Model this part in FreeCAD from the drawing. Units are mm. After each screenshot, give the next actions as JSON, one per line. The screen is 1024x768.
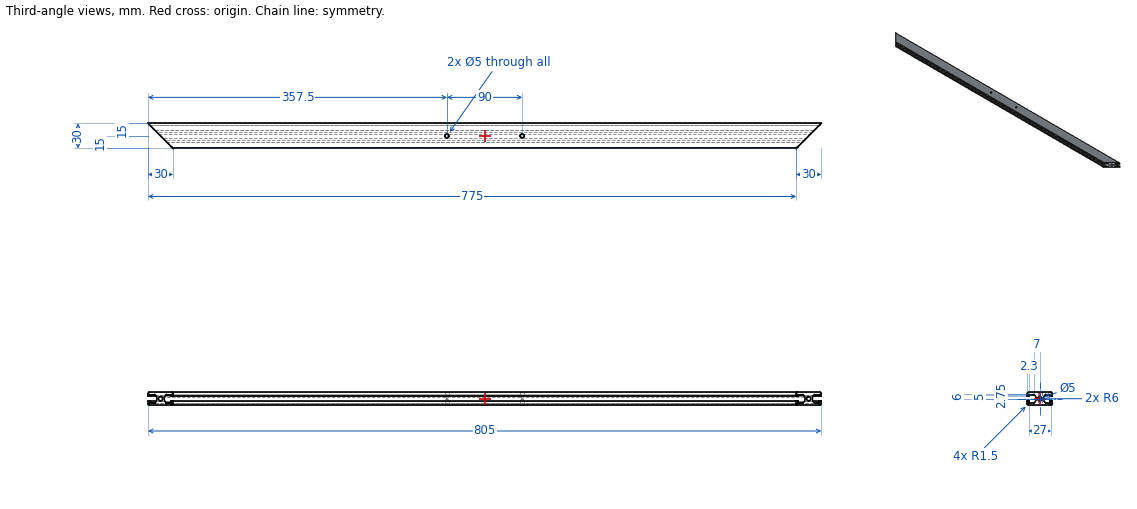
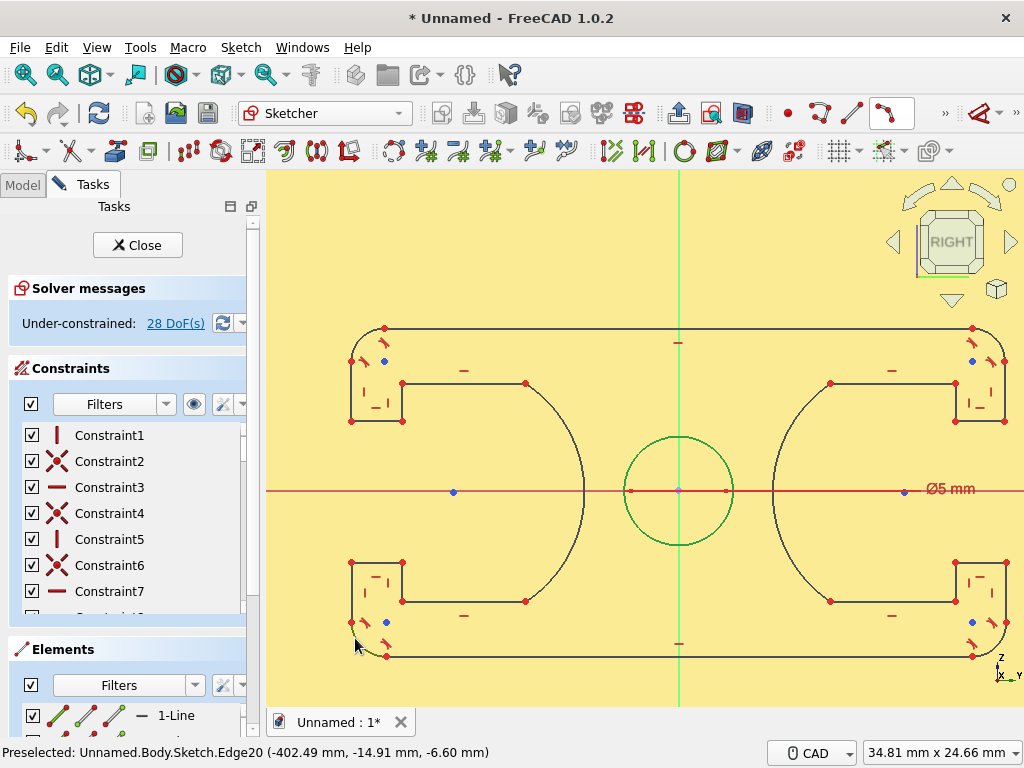
{"action": "scroll", "coordinate": [369, 332], "scroll_direction": "down", "scroll_amount": 2}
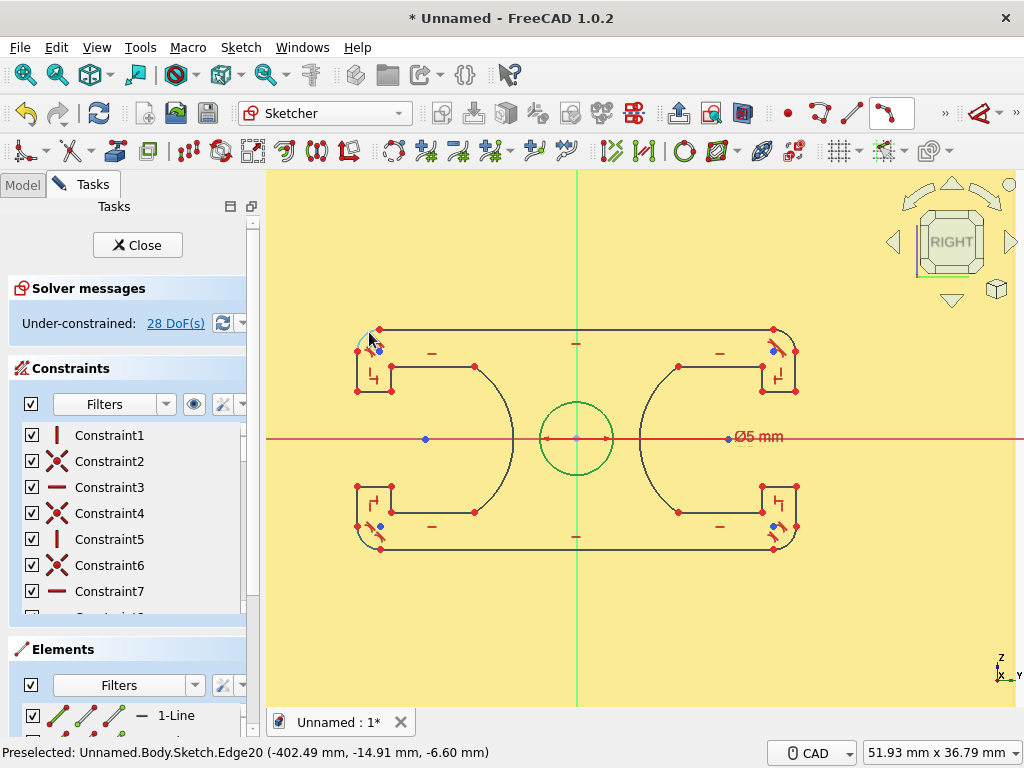
{"action": "scroll", "coordinate": [784, 547], "scroll_direction": "up", "scroll_amount": 2}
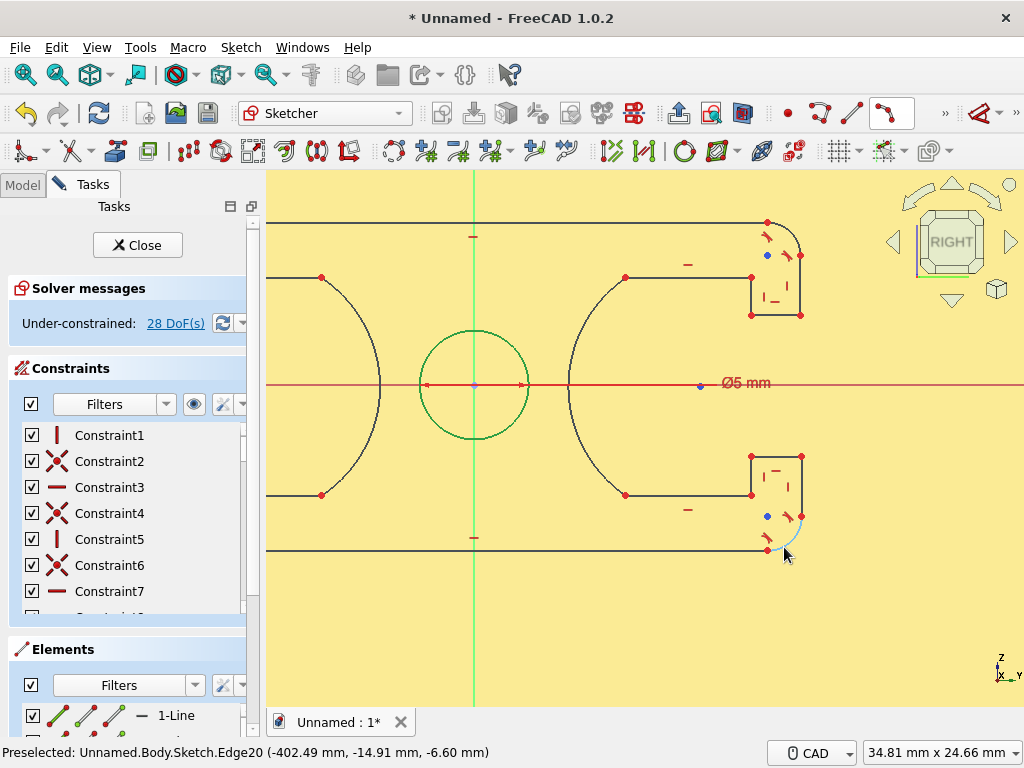
{"action": "left_click", "coordinate": [783, 547]}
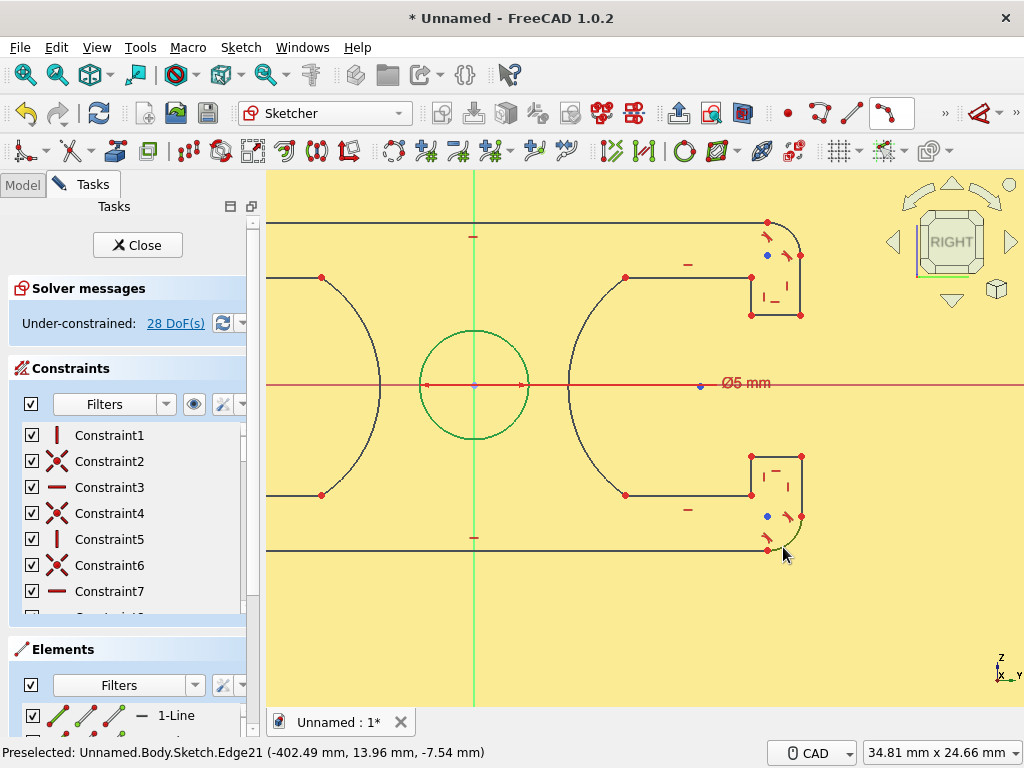
{"action": "left_click", "coordinate": [797, 241]}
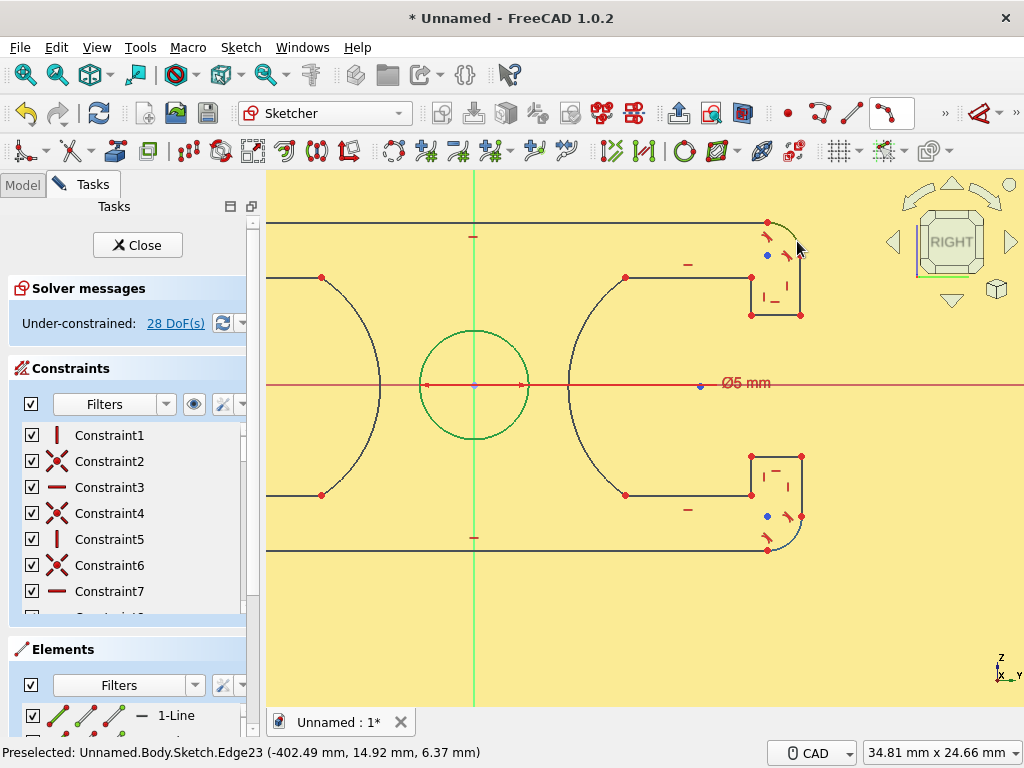
{"action": "scroll", "coordinate": [784, 547], "scroll_direction": "down", "scroll_amount": 2}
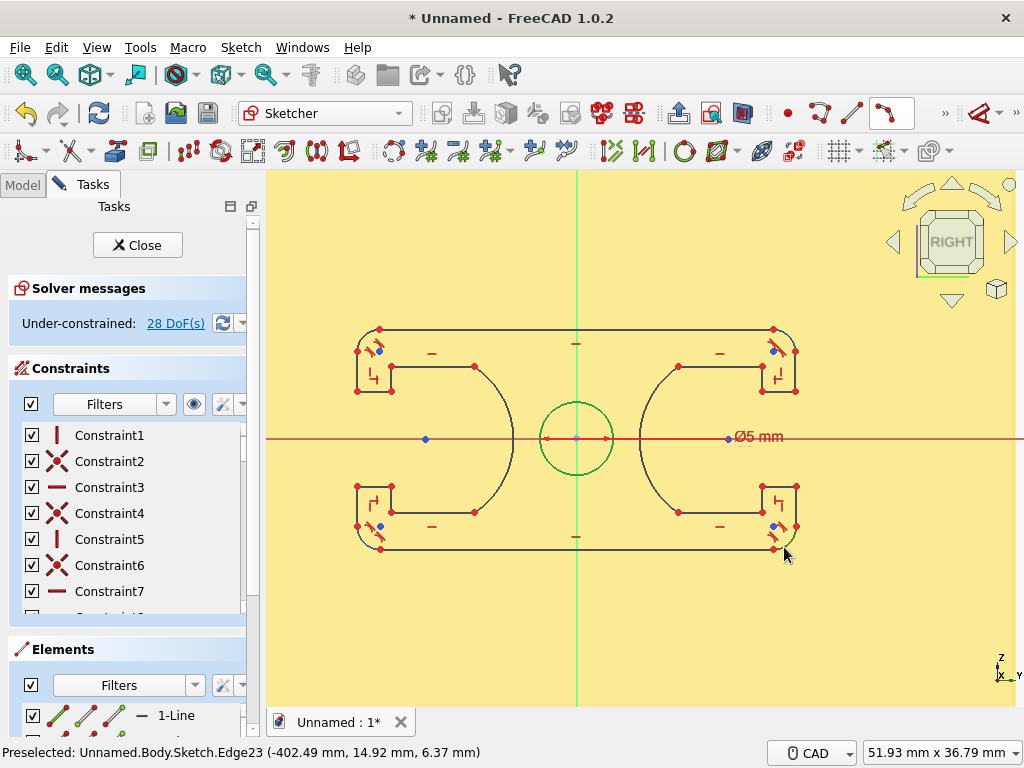
{"action": "scroll", "coordinate": [369, 332], "scroll_direction": "up", "scroll_amount": 2}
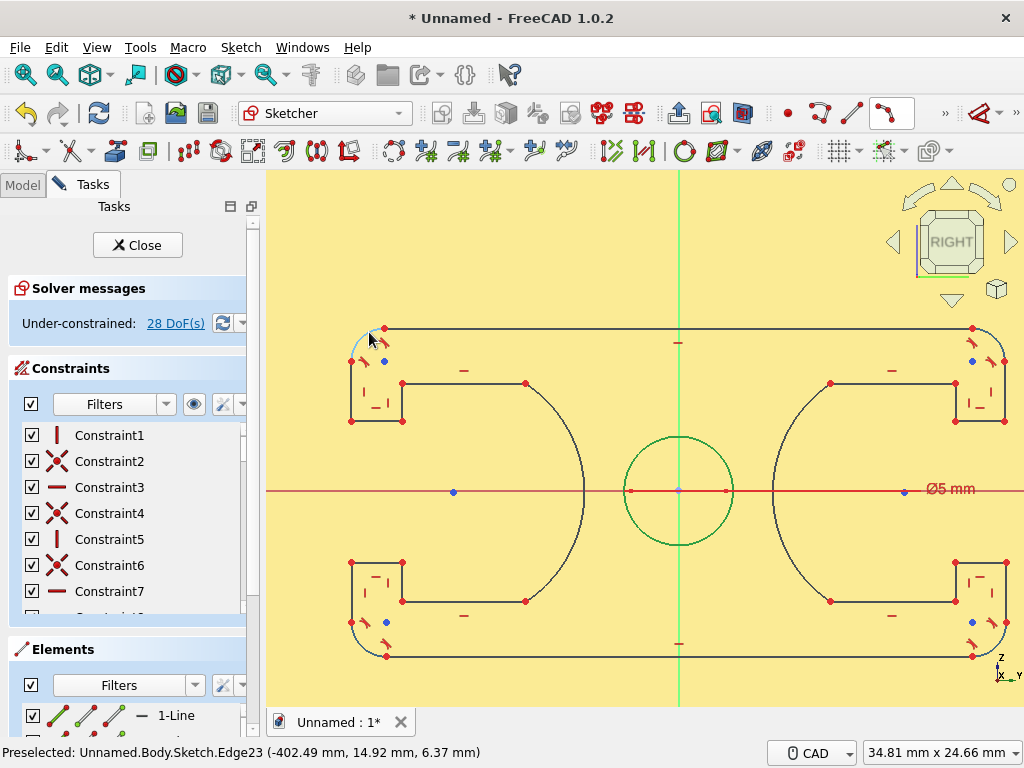
{"action": "left_click", "coordinate": [369, 332]}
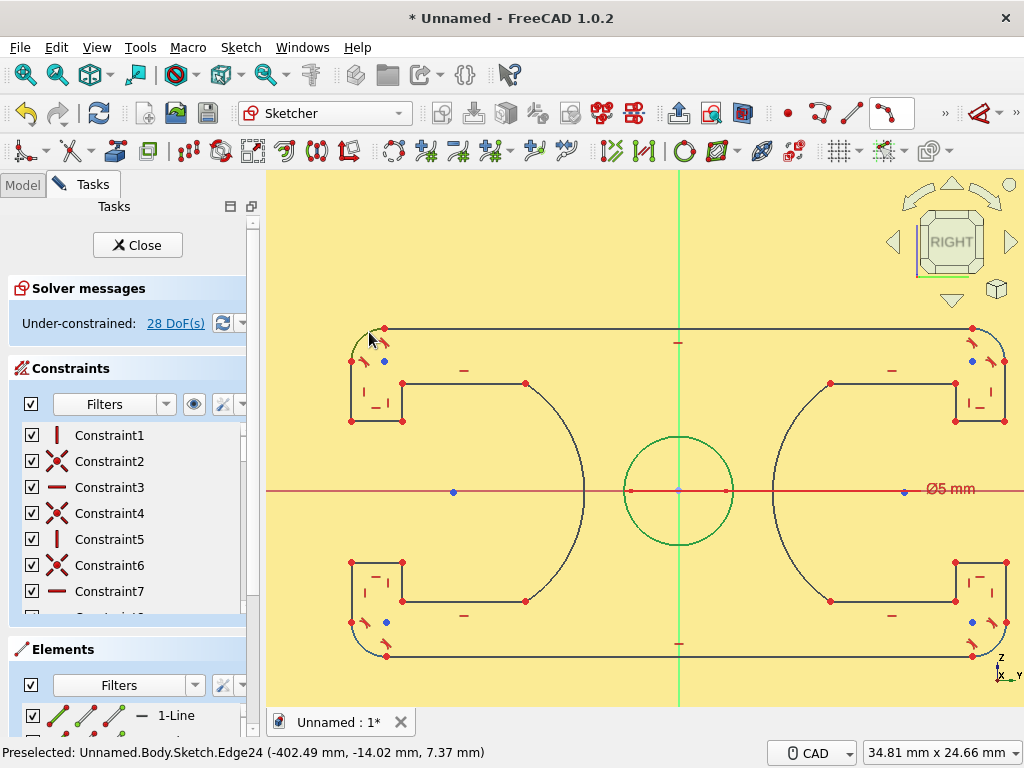
{"action": "key", "text": "e"}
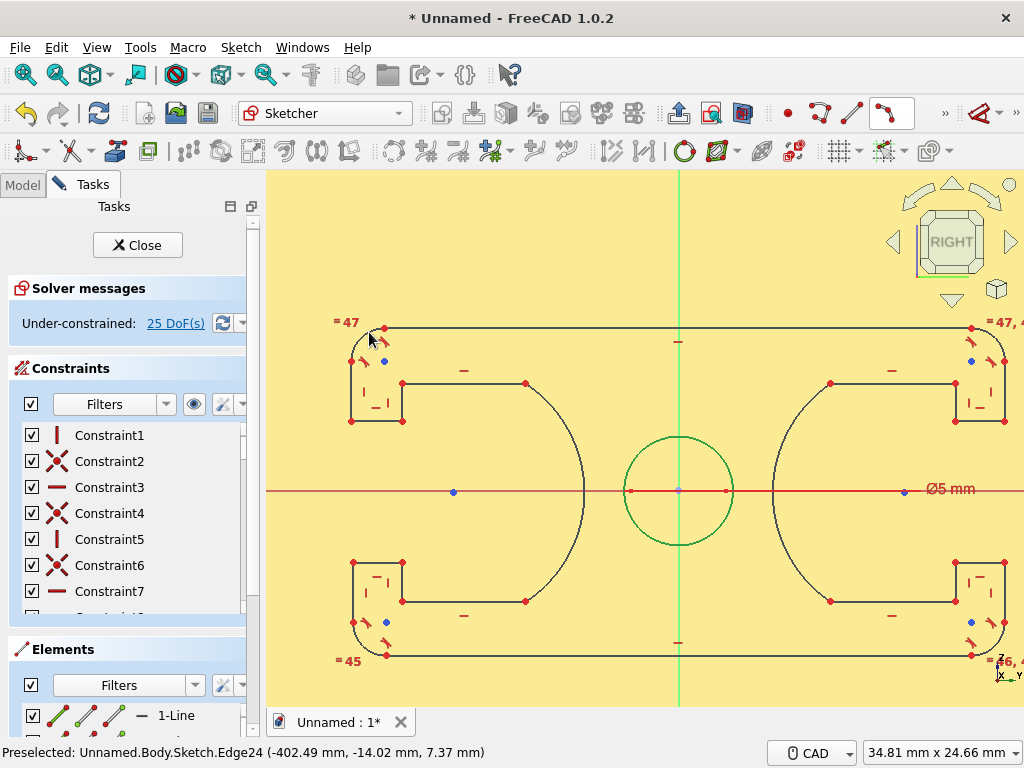
{"action": "left_click", "coordinate": [574, 543]}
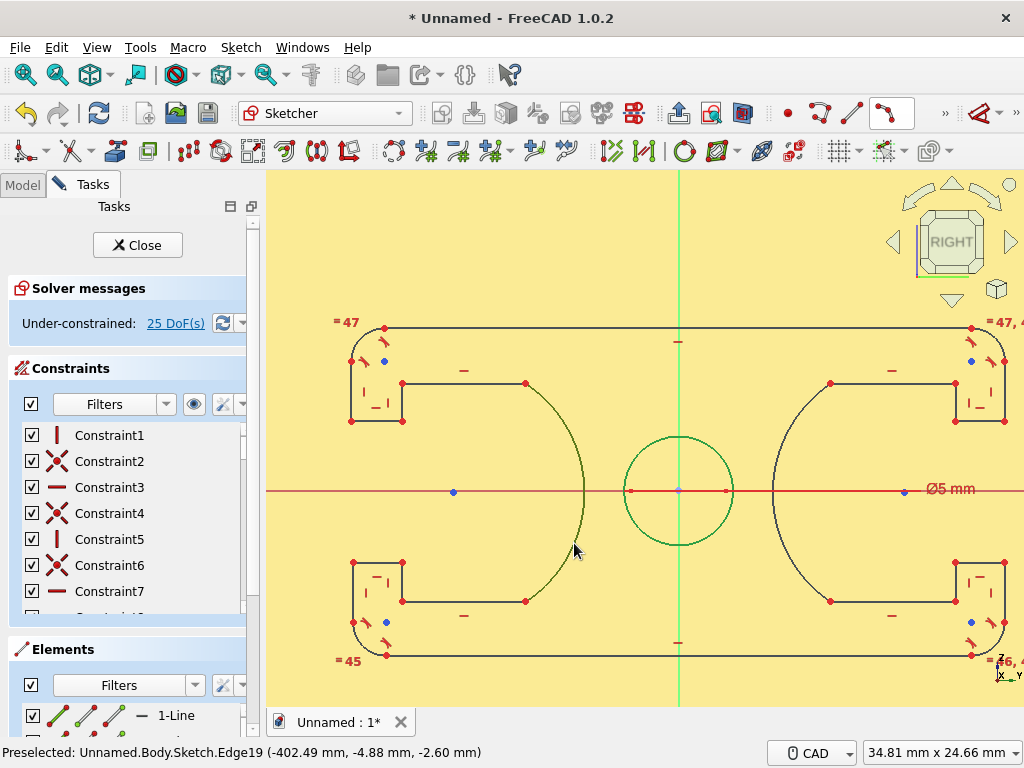
{"action": "left_click", "coordinate": [783, 443]}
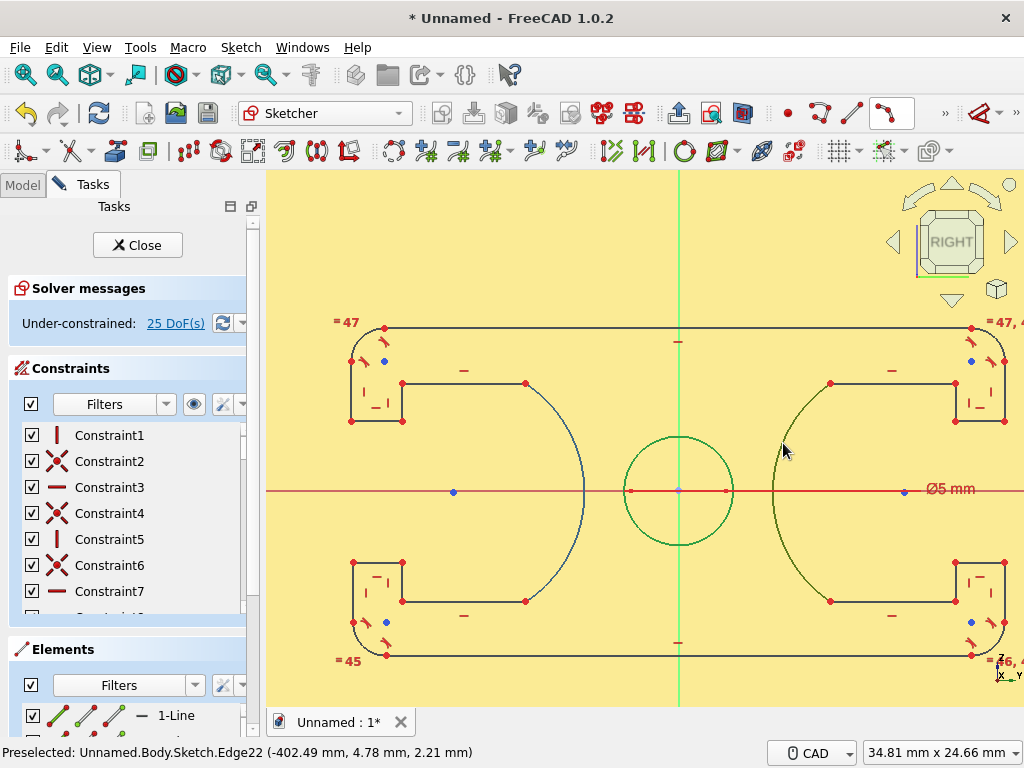
{"action": "key", "text": "e"}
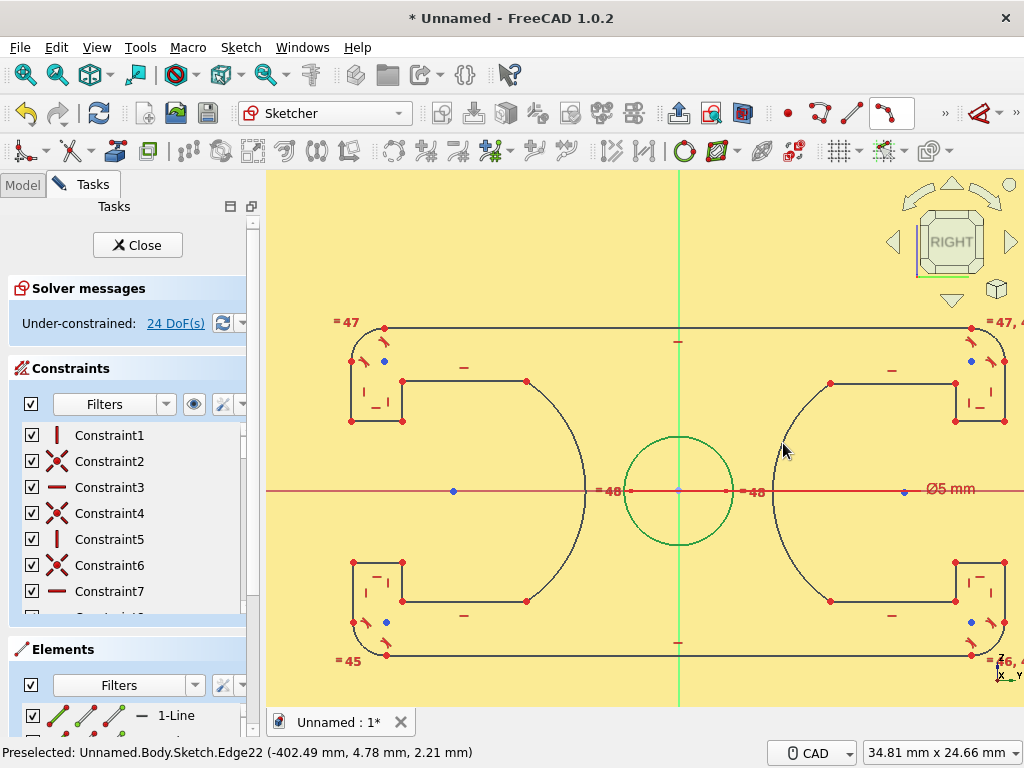
{"action": "left_click", "coordinate": [454, 492]}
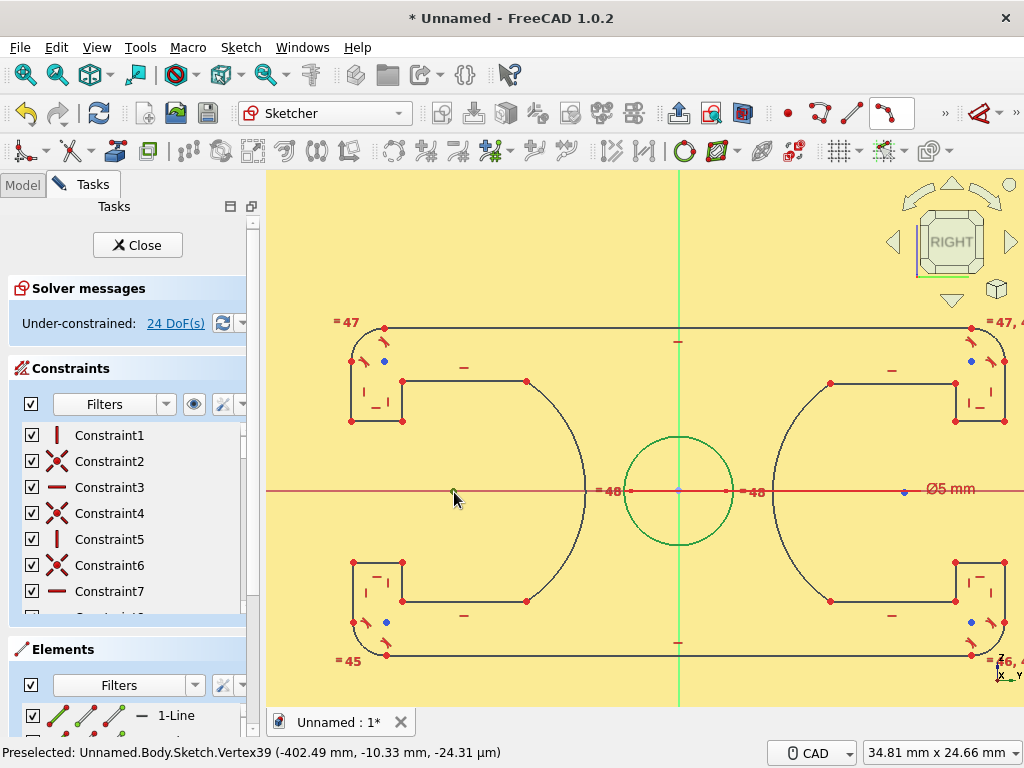
{"action": "left_click", "coordinate": [334, 491]}